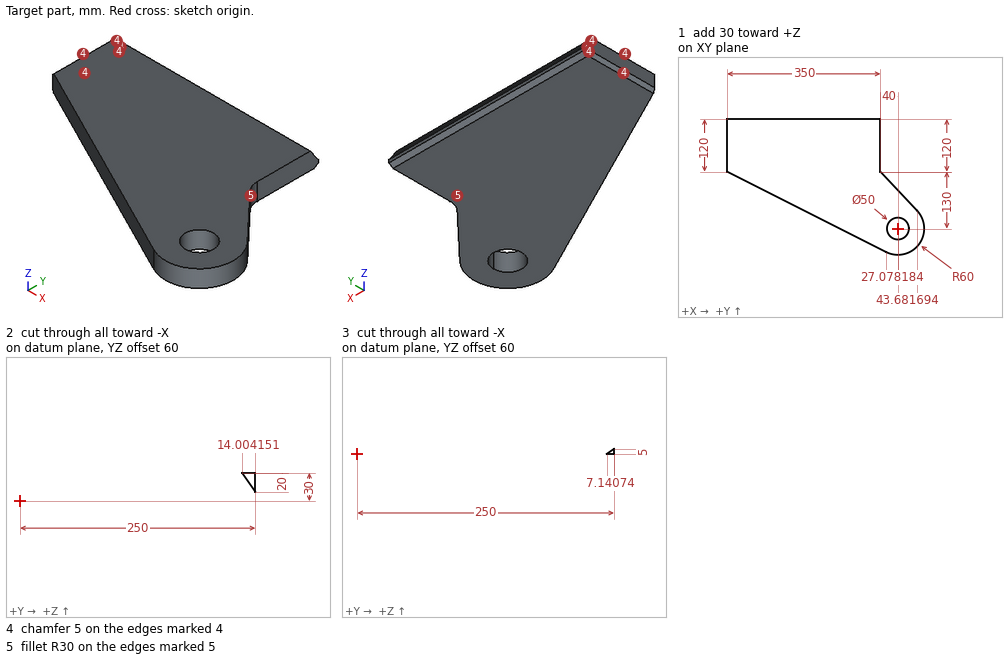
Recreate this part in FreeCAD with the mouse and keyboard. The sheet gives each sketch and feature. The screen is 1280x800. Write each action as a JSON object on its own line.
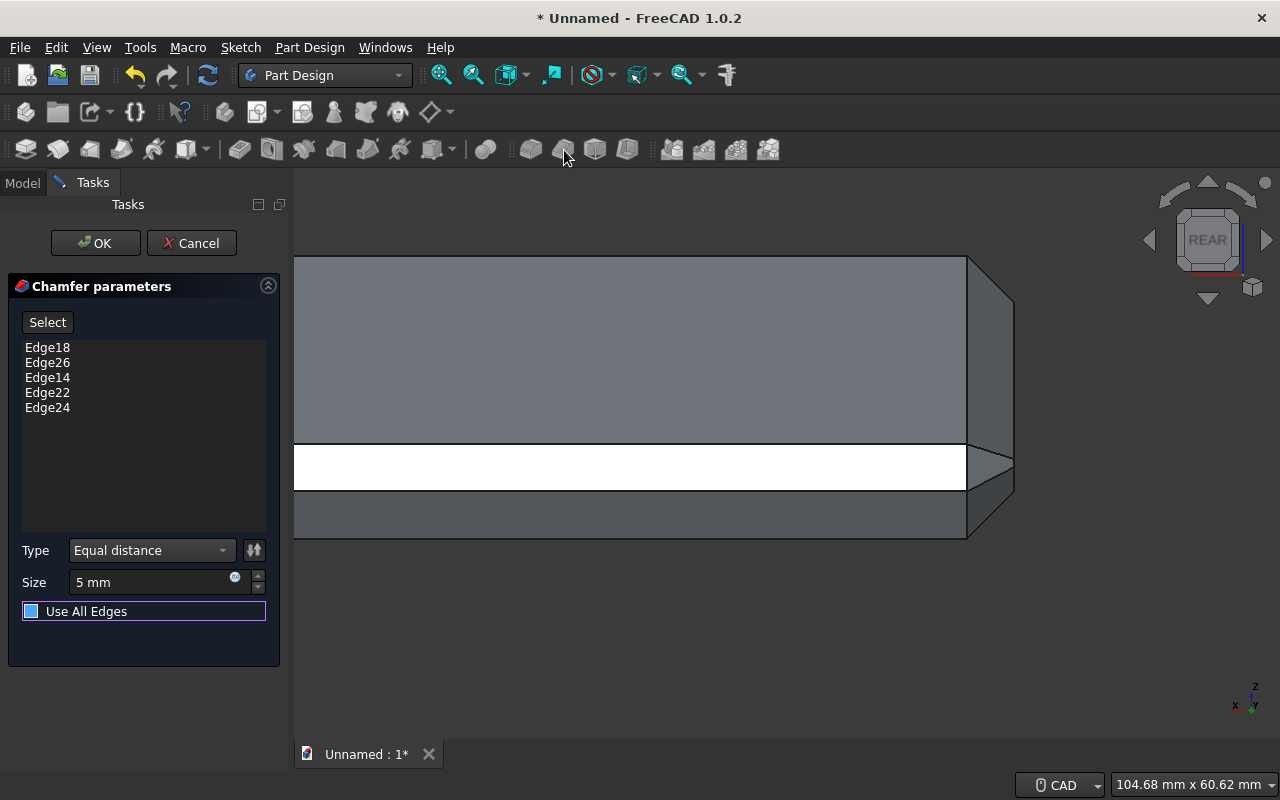
{"action": "left_click", "coordinate": [96, 243]}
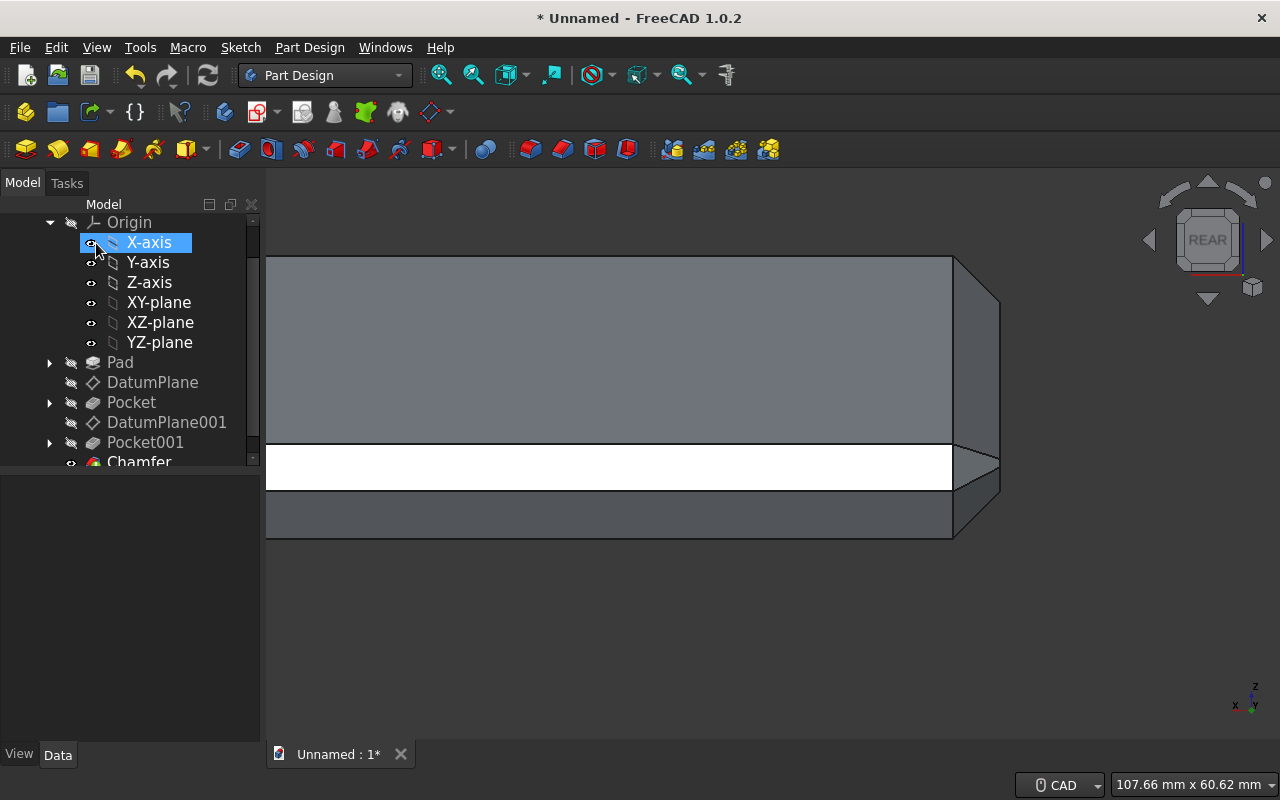
{"action": "left_click", "coordinate": [442, 76]}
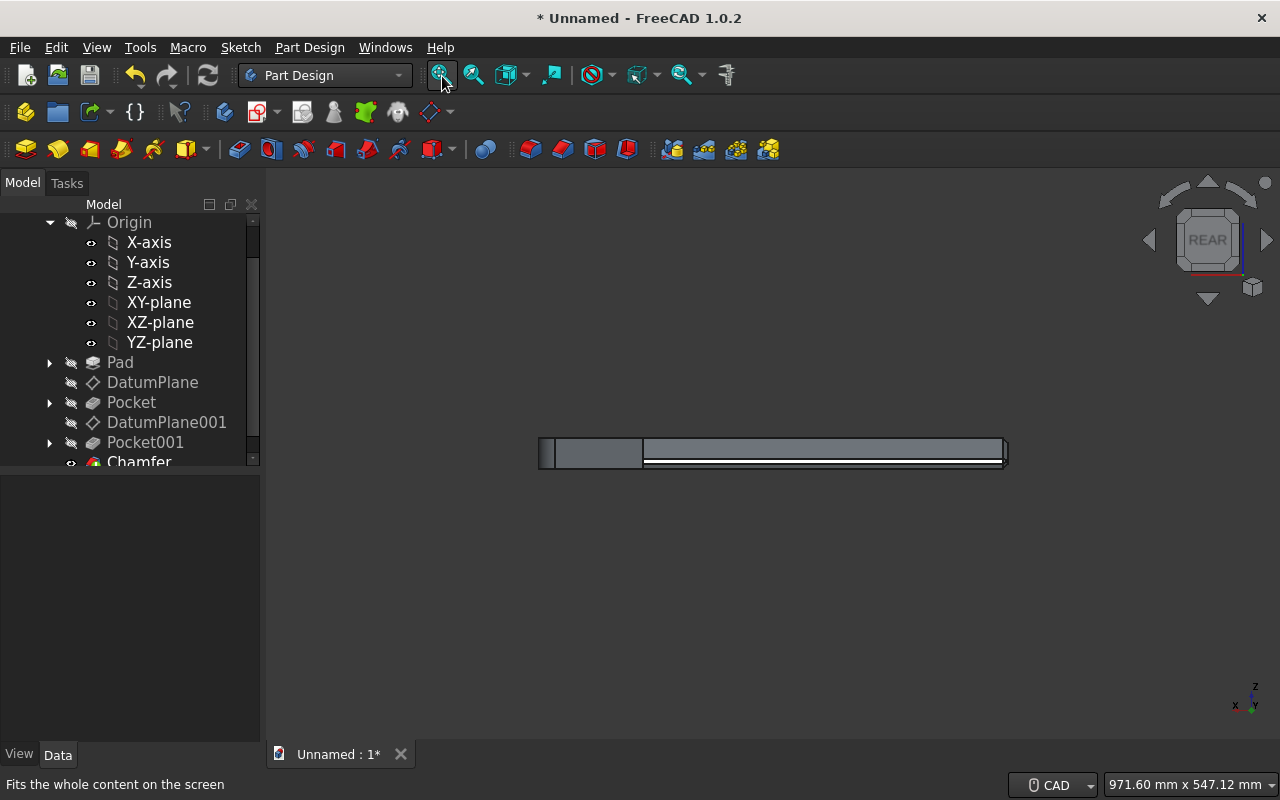
{"action": "key", "text": "0"}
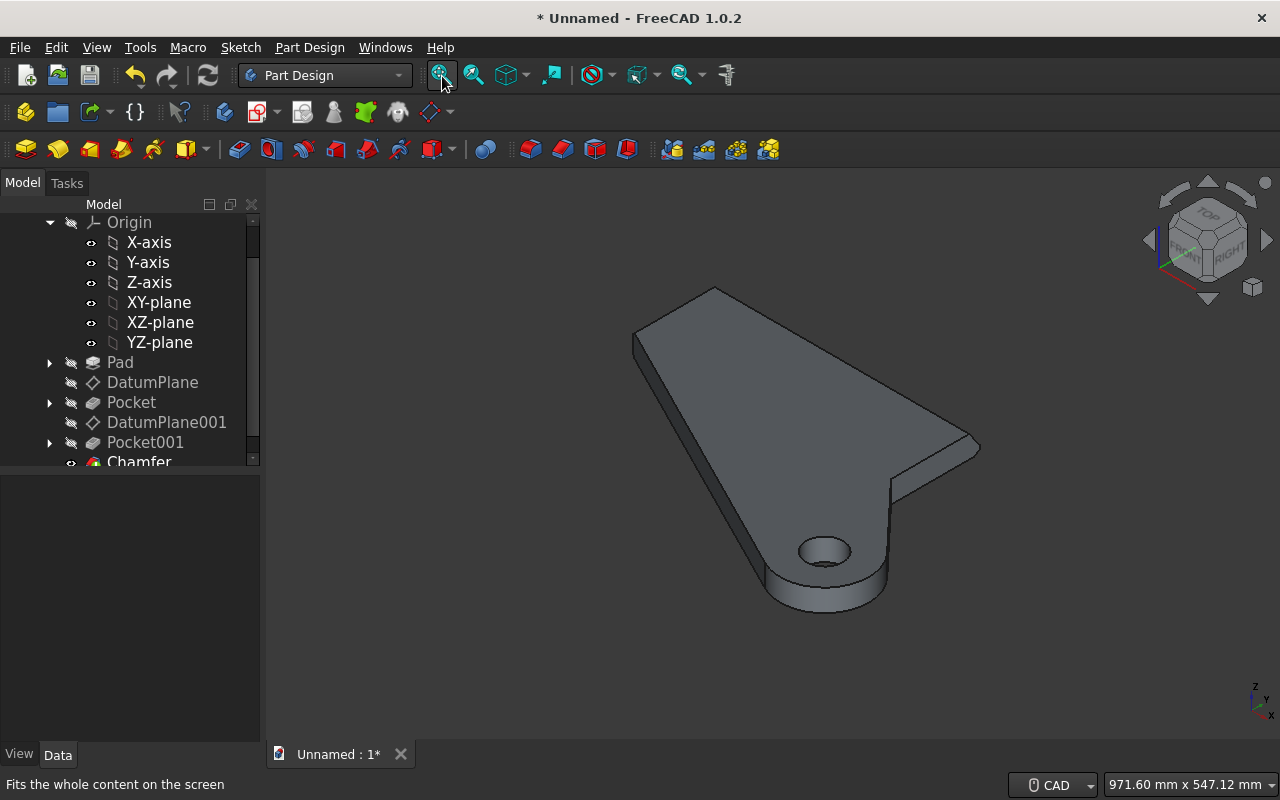
{"action": "key", "text": "2"}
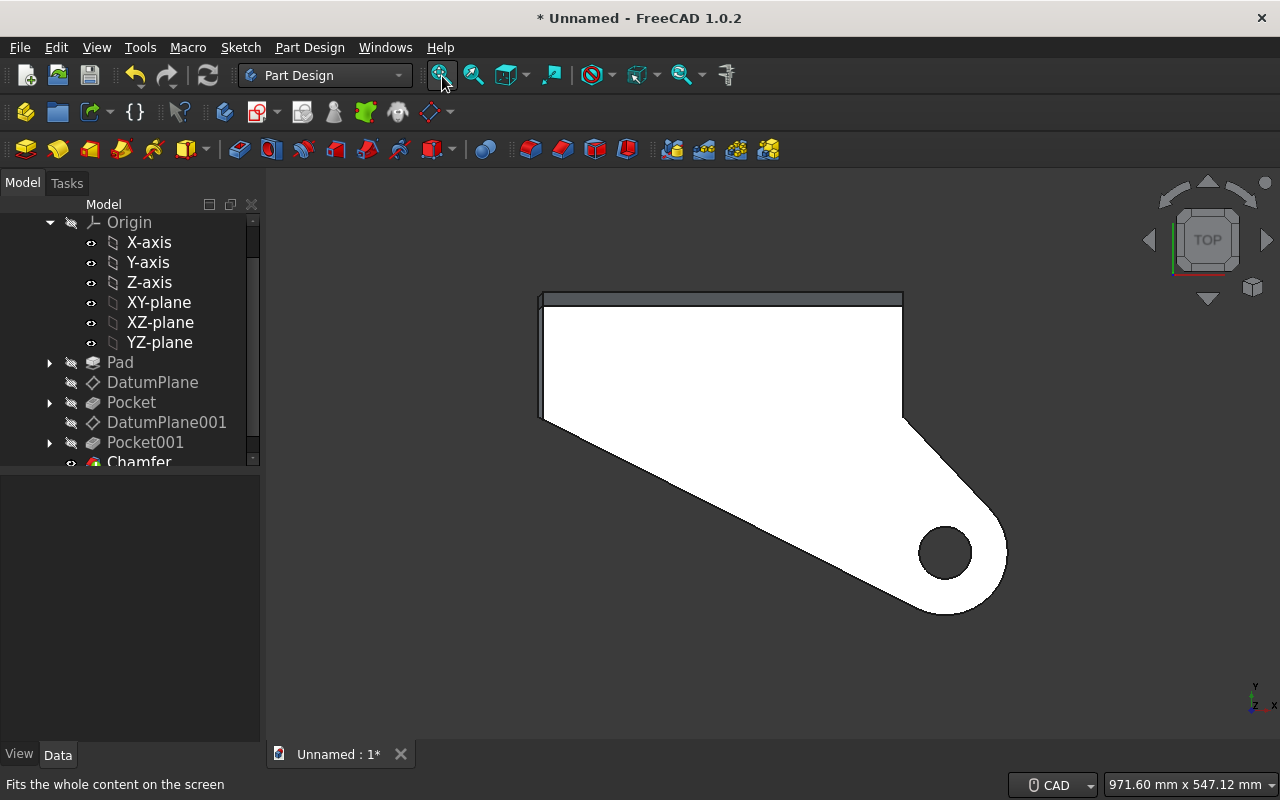
{"action": "key", "text": "1"}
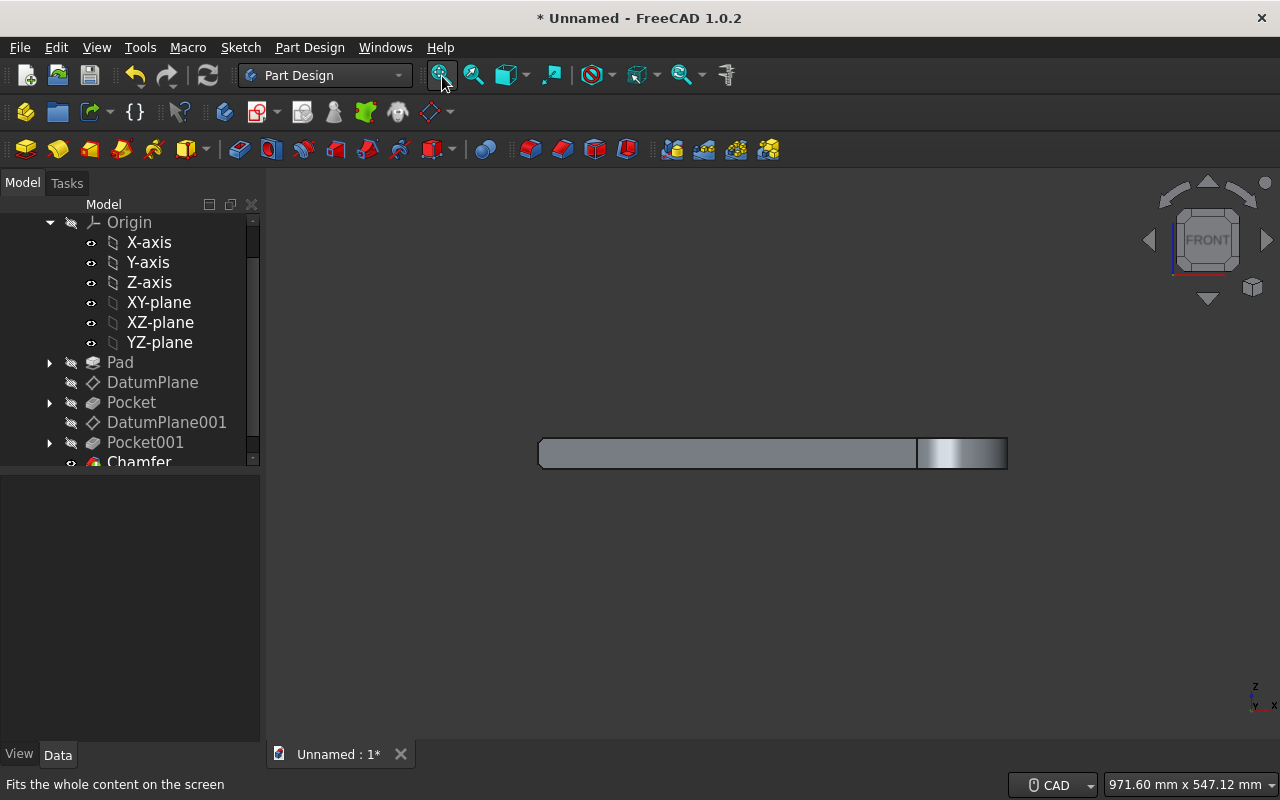
{"action": "key", "text": "3"}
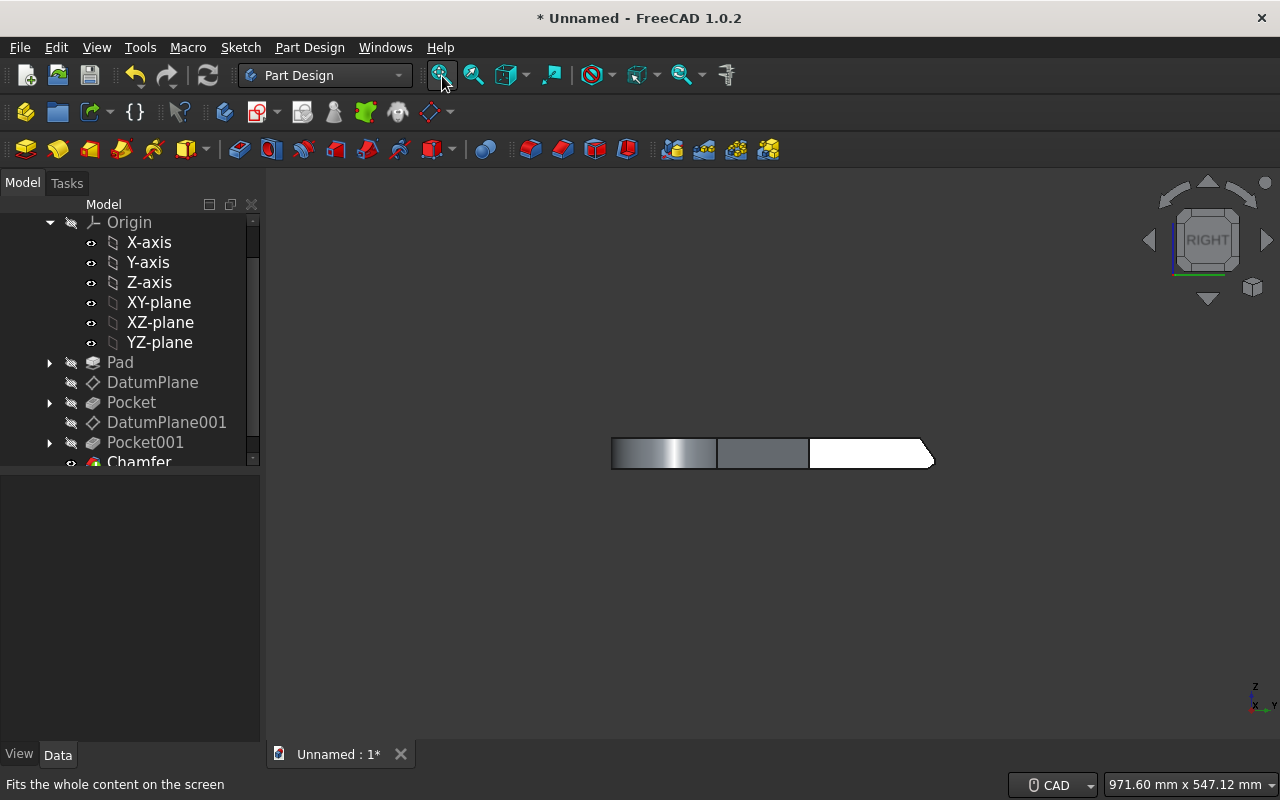
{"action": "key", "text": "v f"}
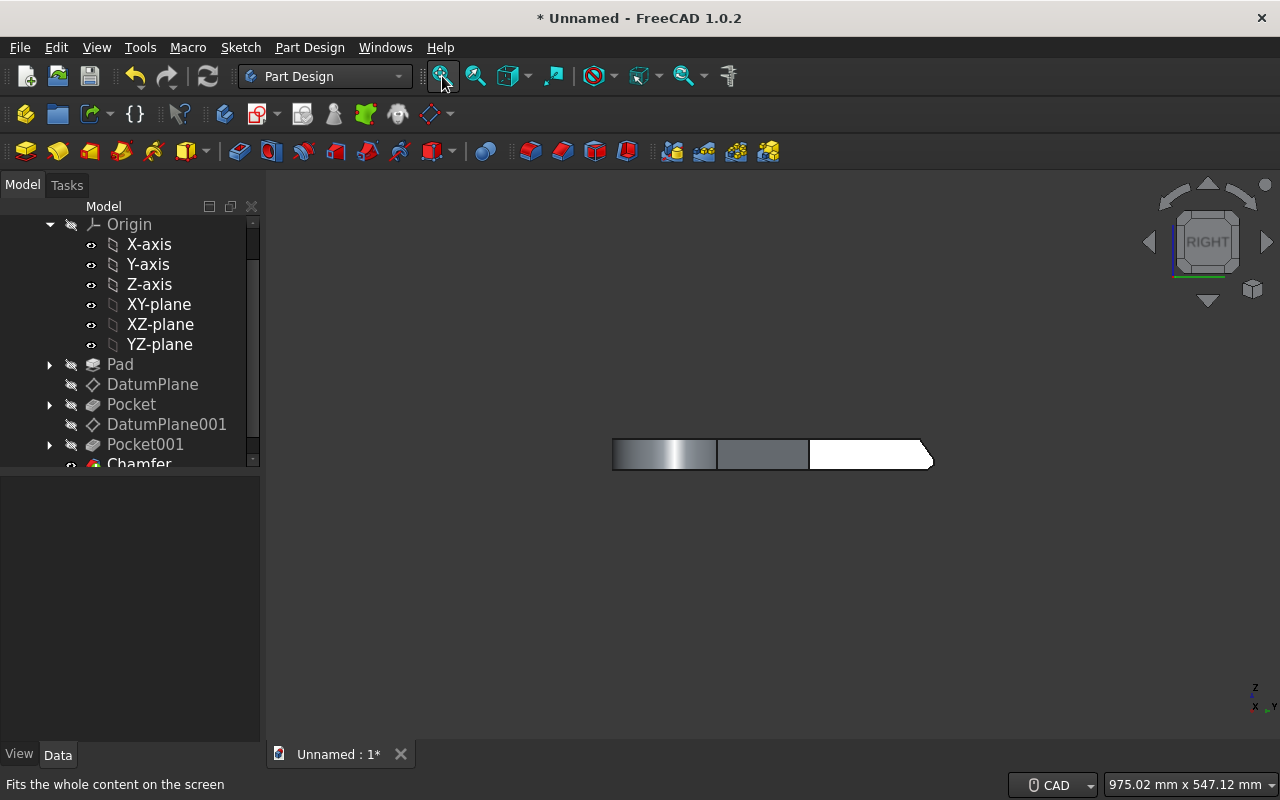
{"action": "key", "text": "5"}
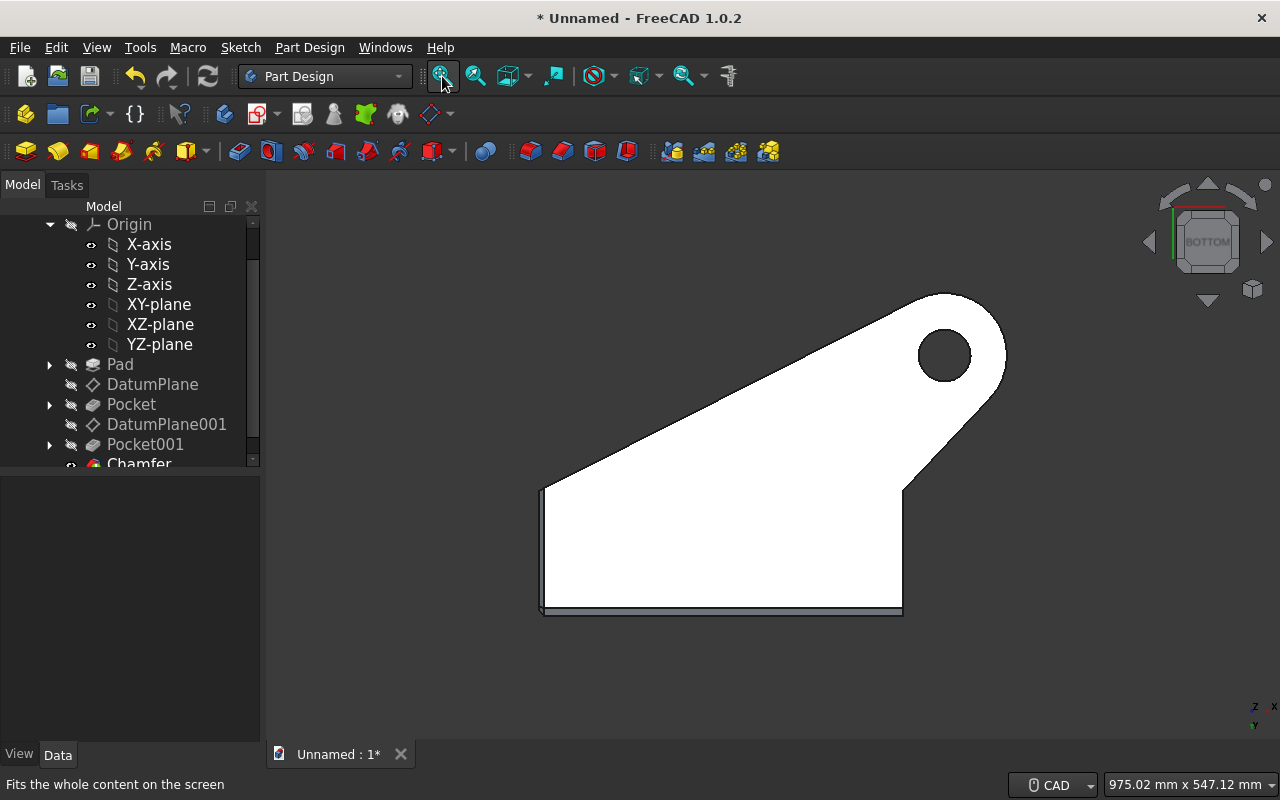
{"action": "key", "text": "4"}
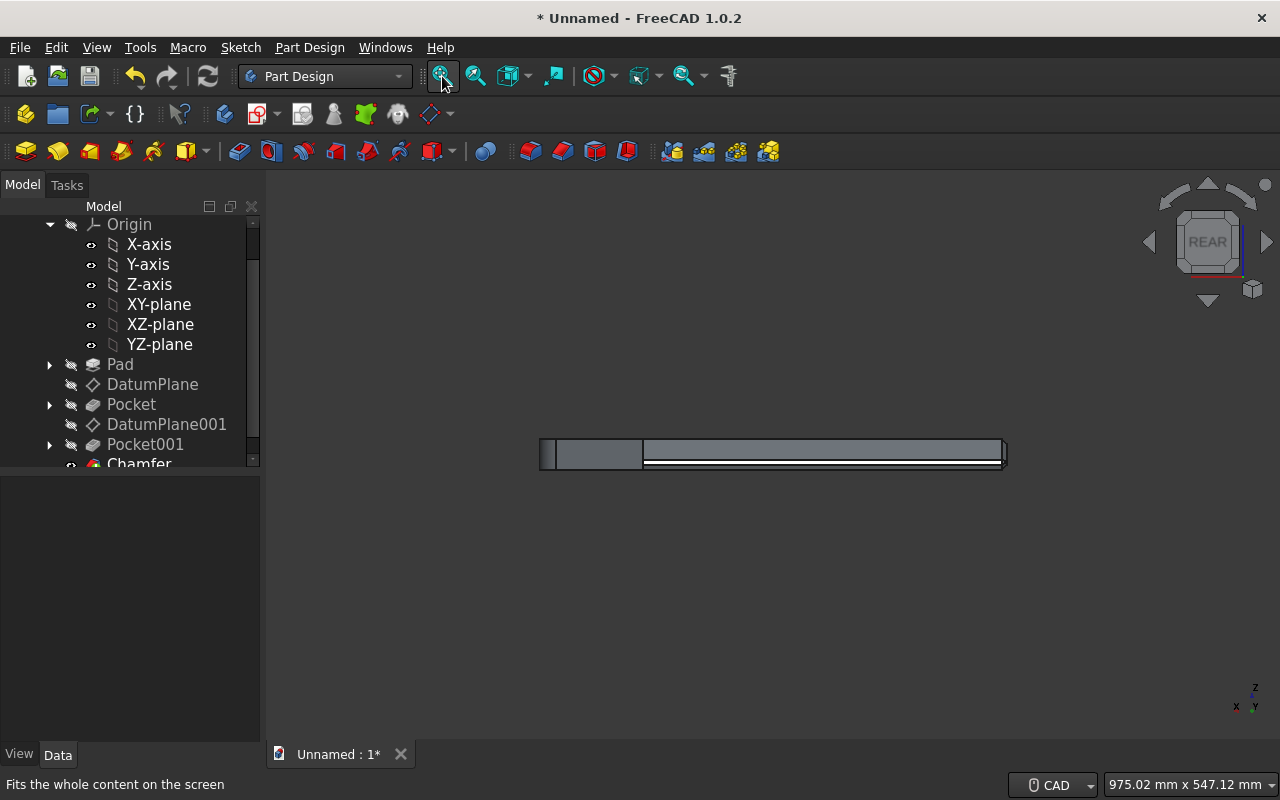
{"action": "key", "text": "6"}